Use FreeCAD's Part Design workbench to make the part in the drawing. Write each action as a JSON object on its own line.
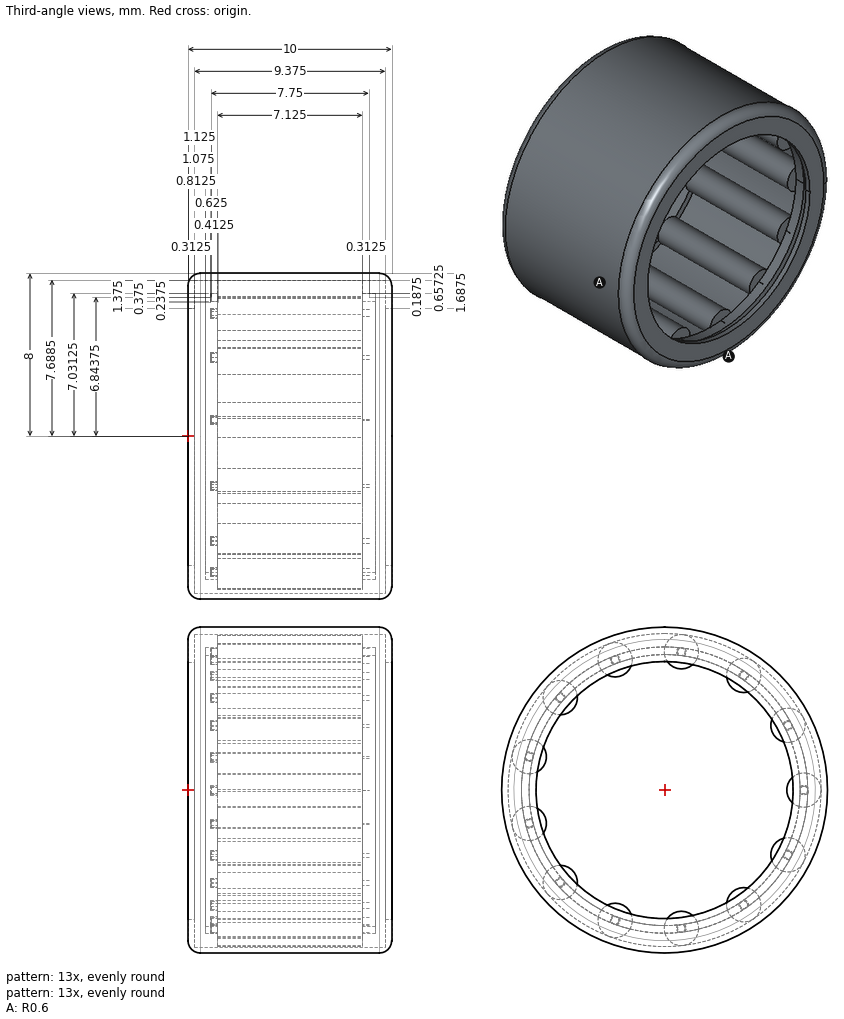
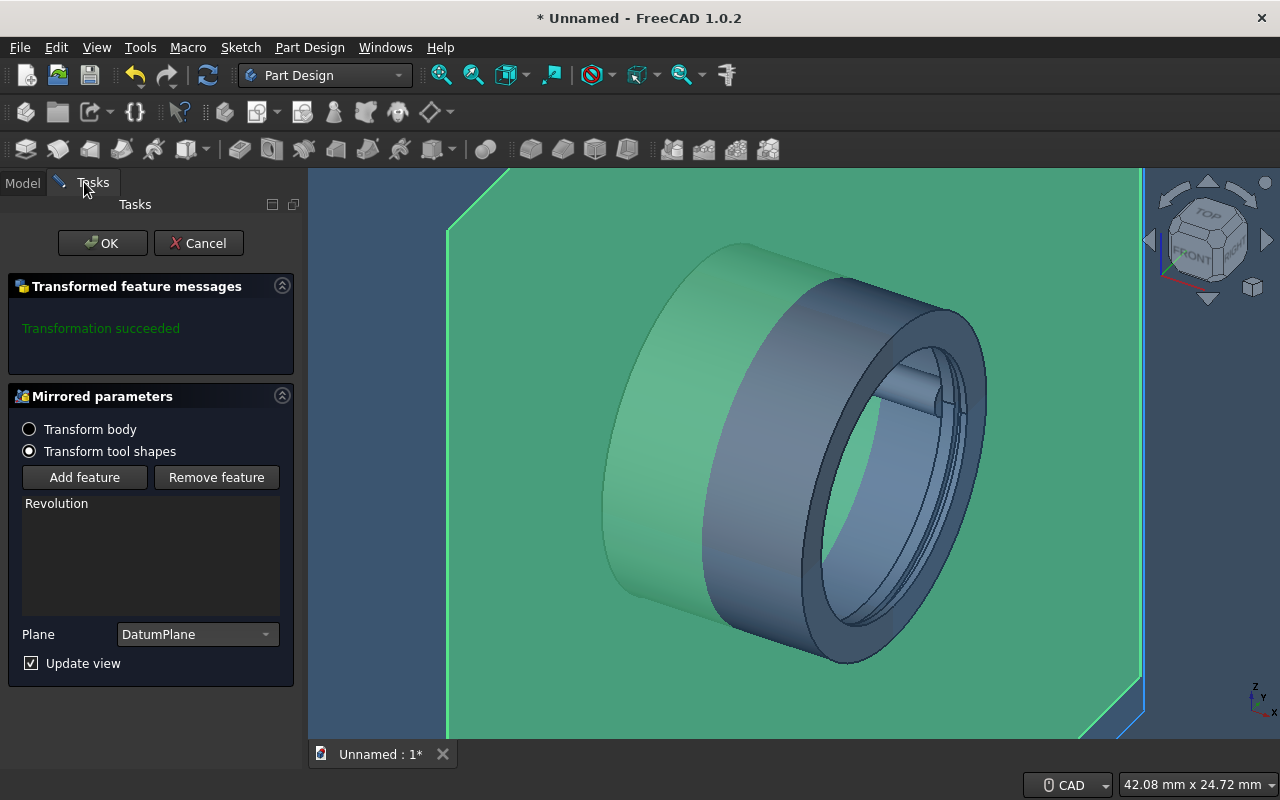
{"action": "left_click", "coordinate": [103, 243]}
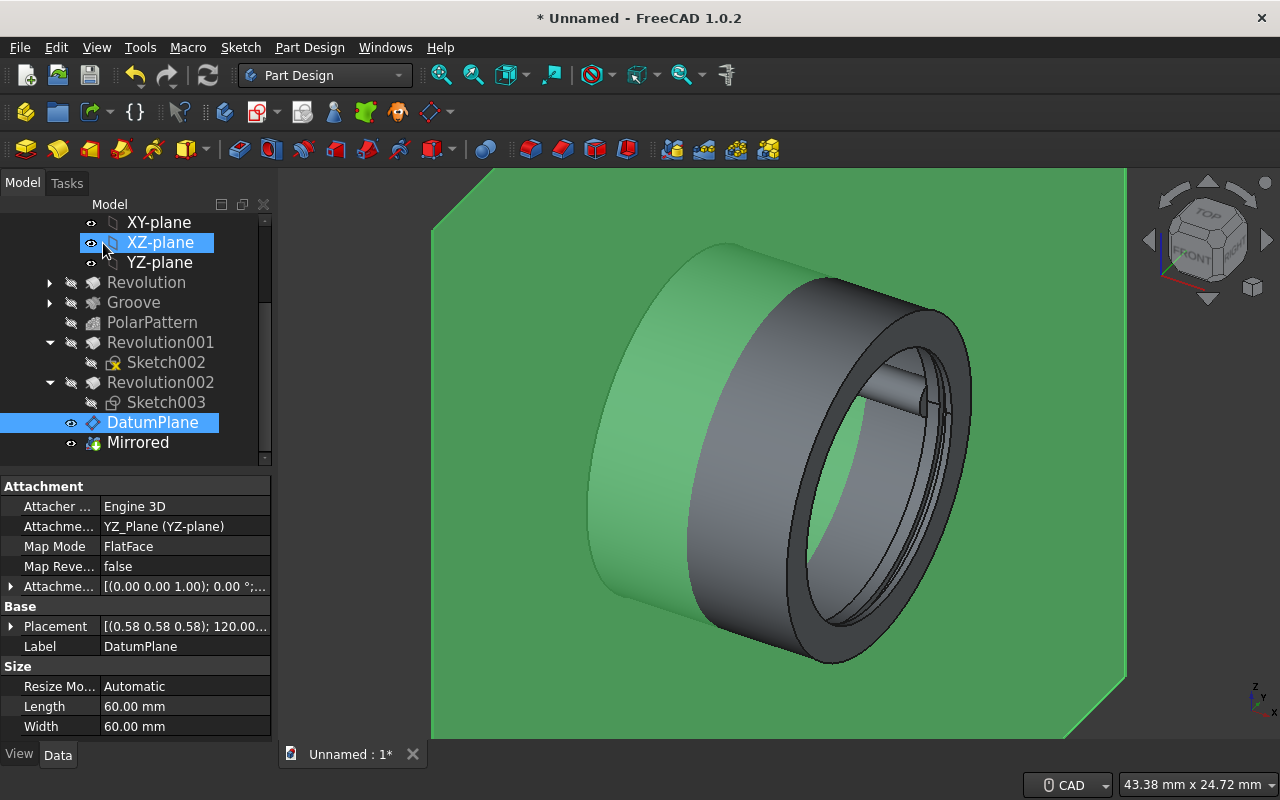
{"action": "left_click", "coordinate": [116, 423]}
{"action": "key", "text": "space"}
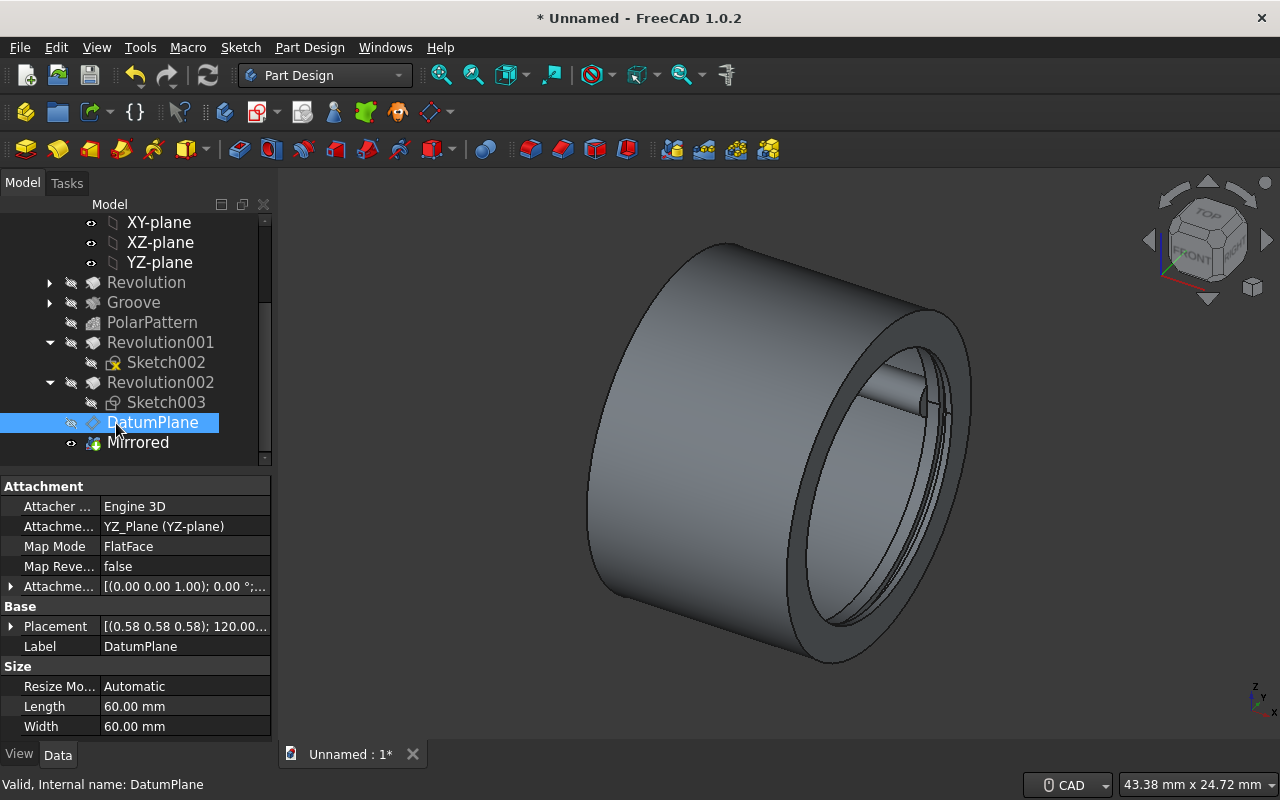
{"action": "left_click", "coordinate": [116, 343]}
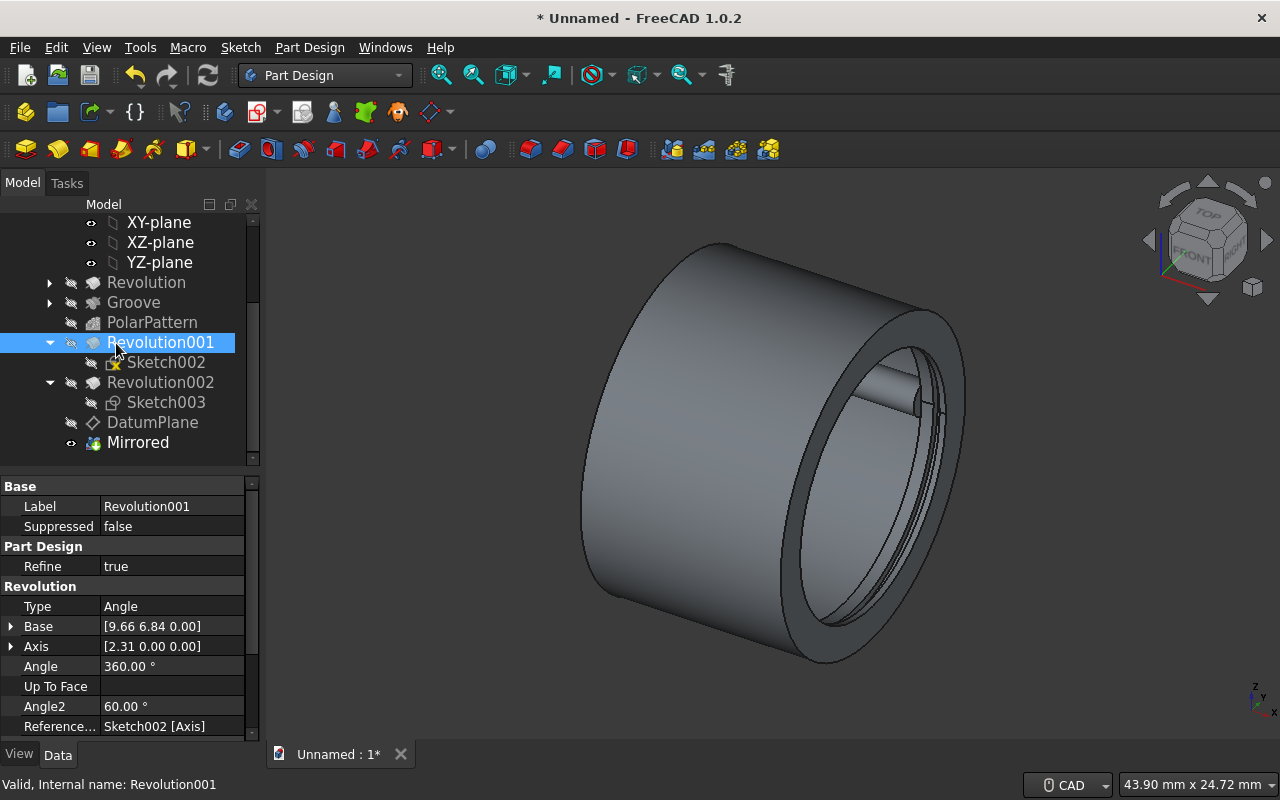
{"action": "left_click", "coordinate": [736, 150]}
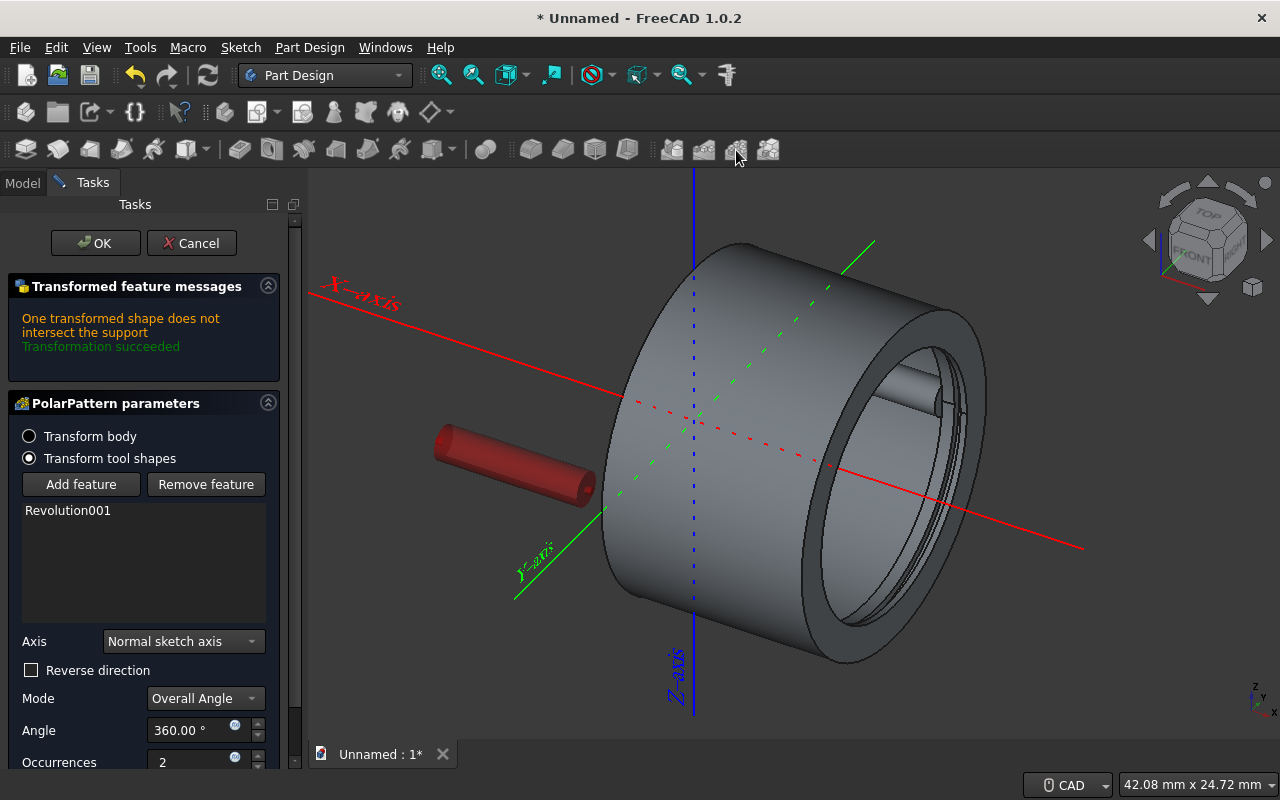
{"action": "left_click", "coordinate": [184, 642]}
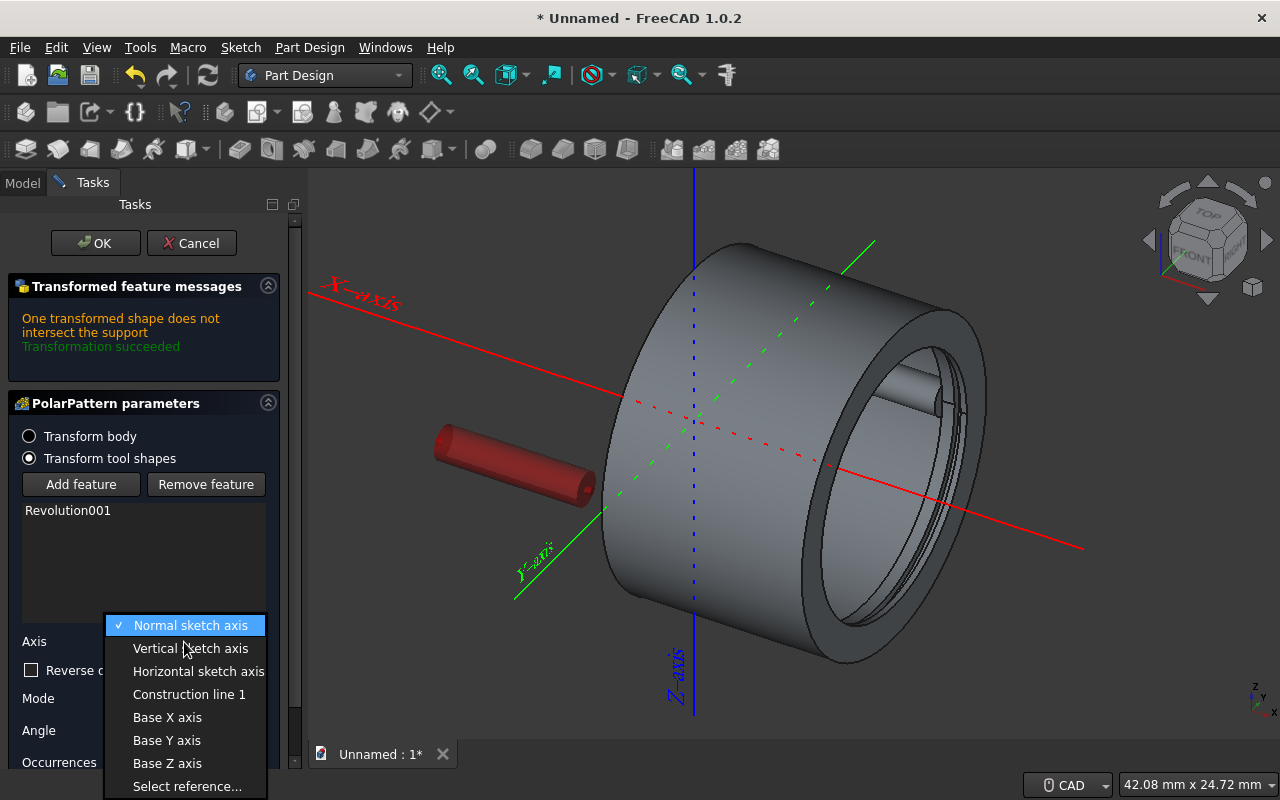
{"action": "left_click", "coordinate": [184, 718]}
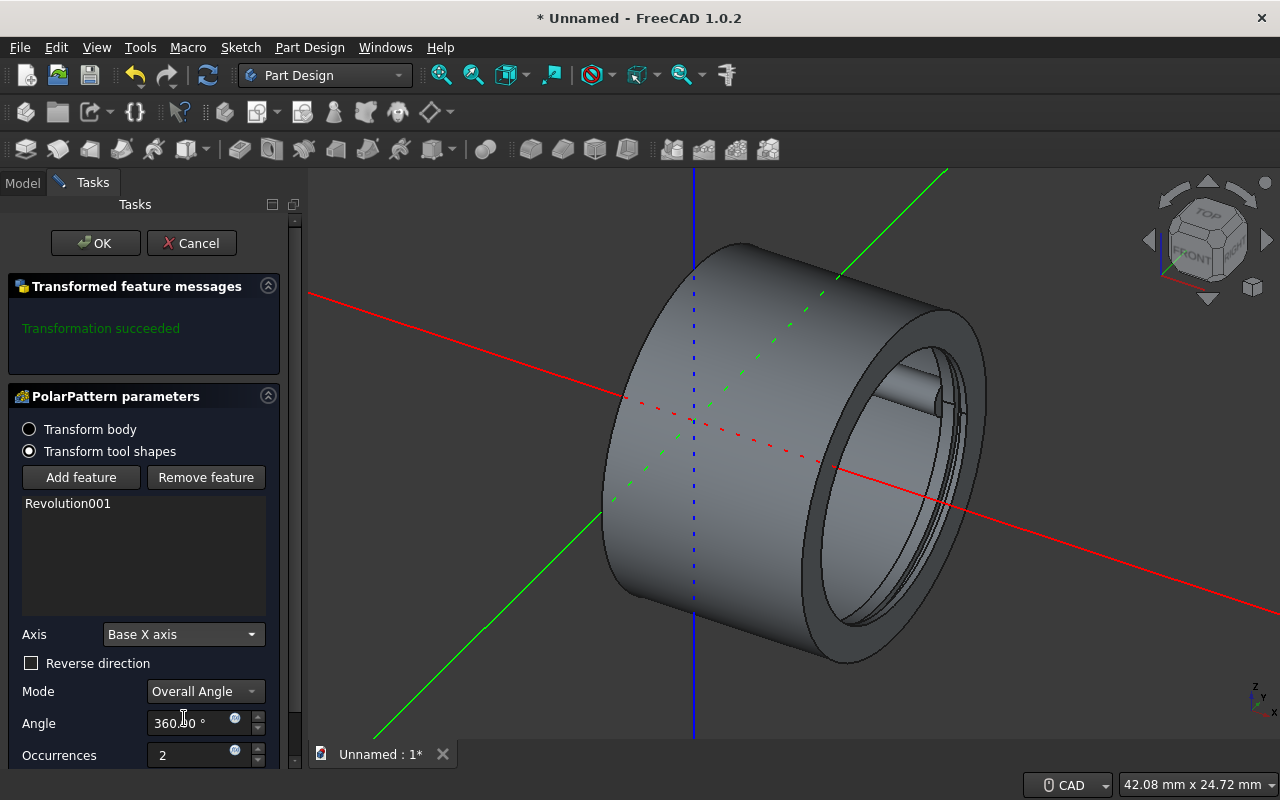
{"action": "triple_click", "coordinate": [198, 755]}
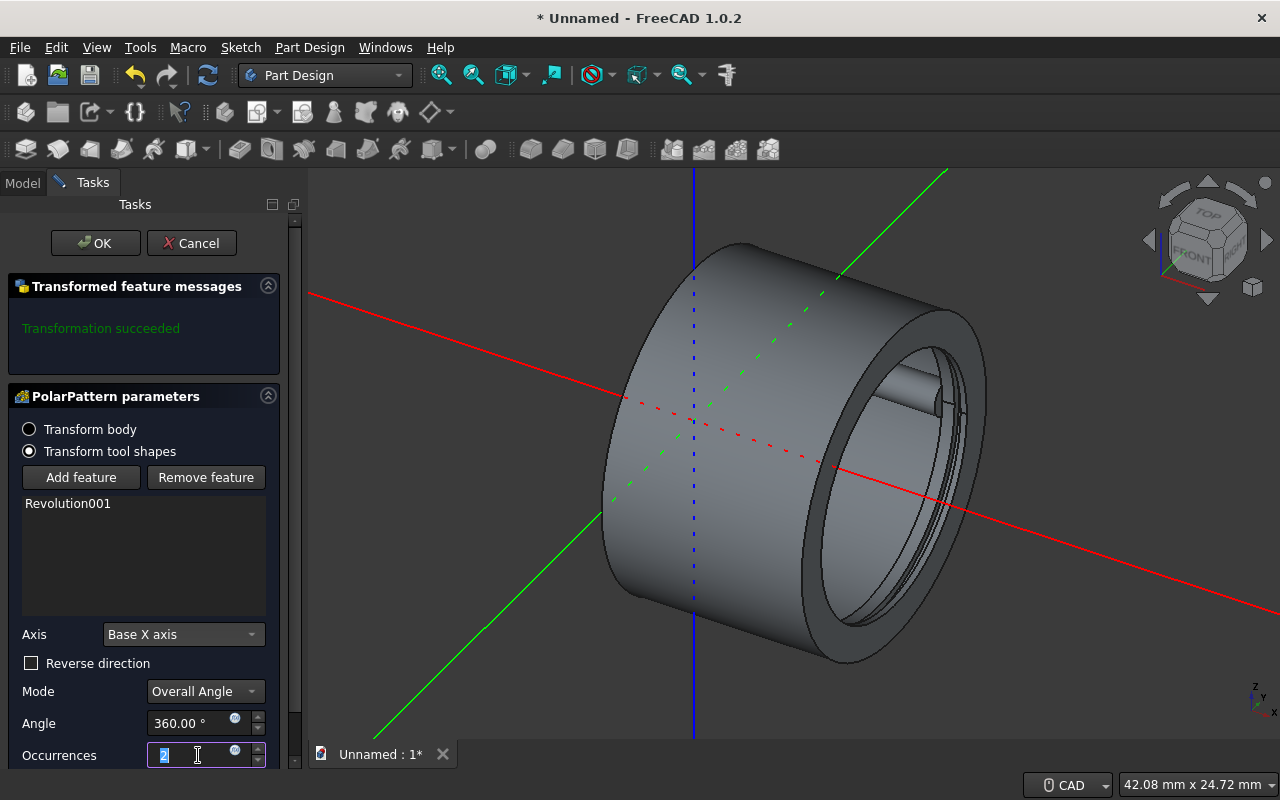
{"action": "type", "text": "13"}
{"action": "key", "text": "Tab"}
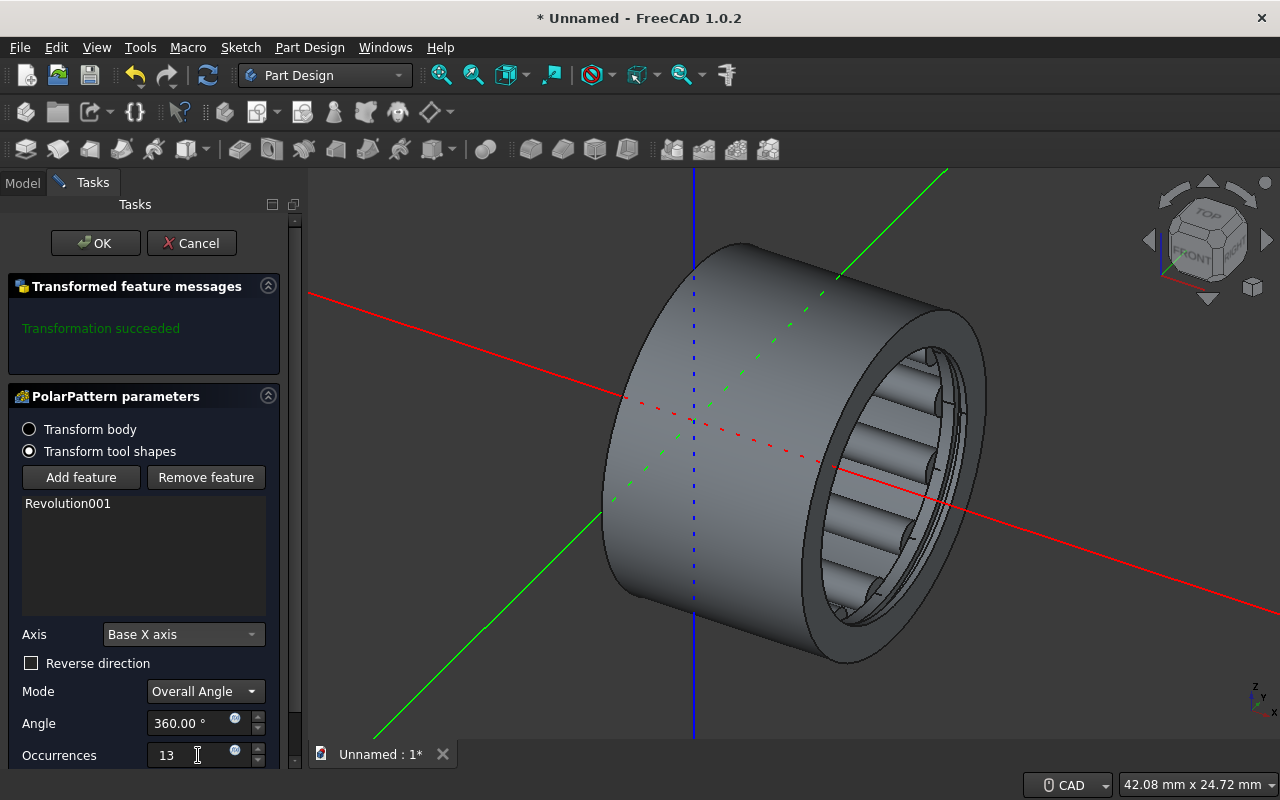
{"action": "left_click", "coordinate": [96, 243]}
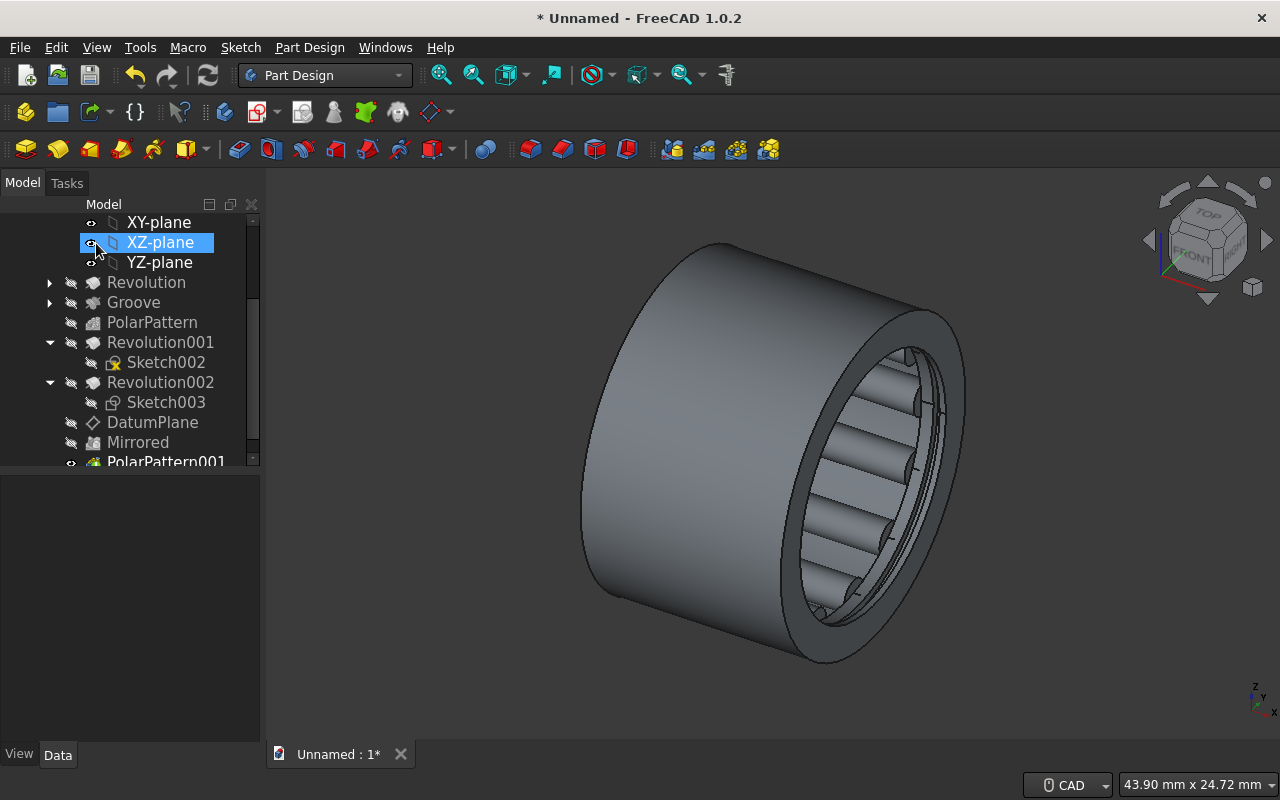
{"action": "left_click", "coordinate": [781, 577]}